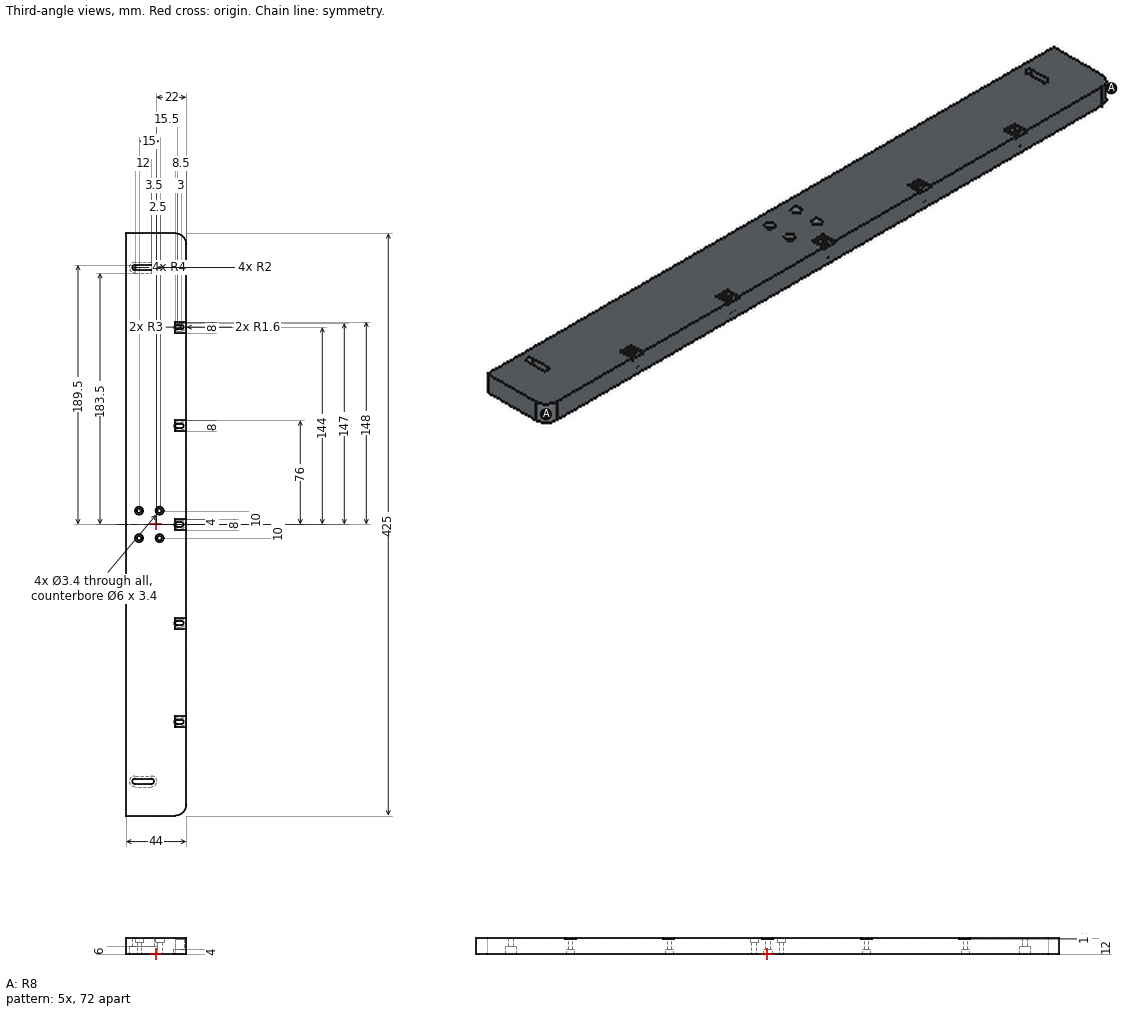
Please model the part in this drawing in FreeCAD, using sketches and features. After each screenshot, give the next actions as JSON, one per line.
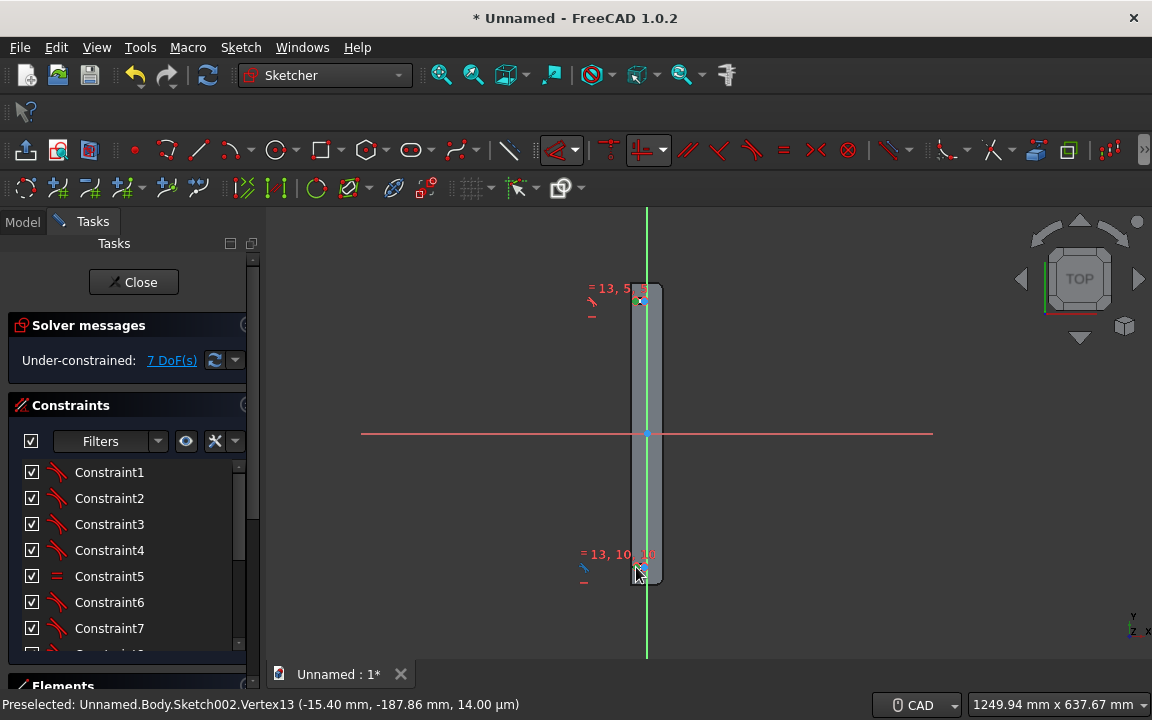
{"action": "left_click", "coordinate": [393, 434]}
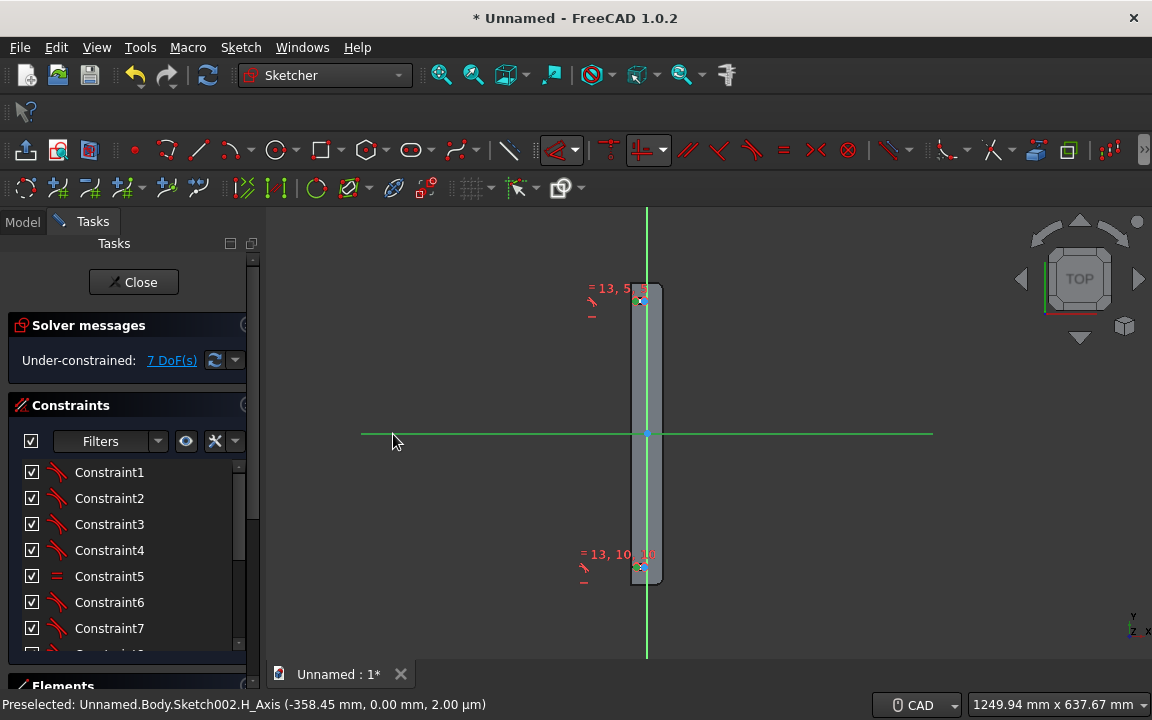
{"action": "key", "text": "s"}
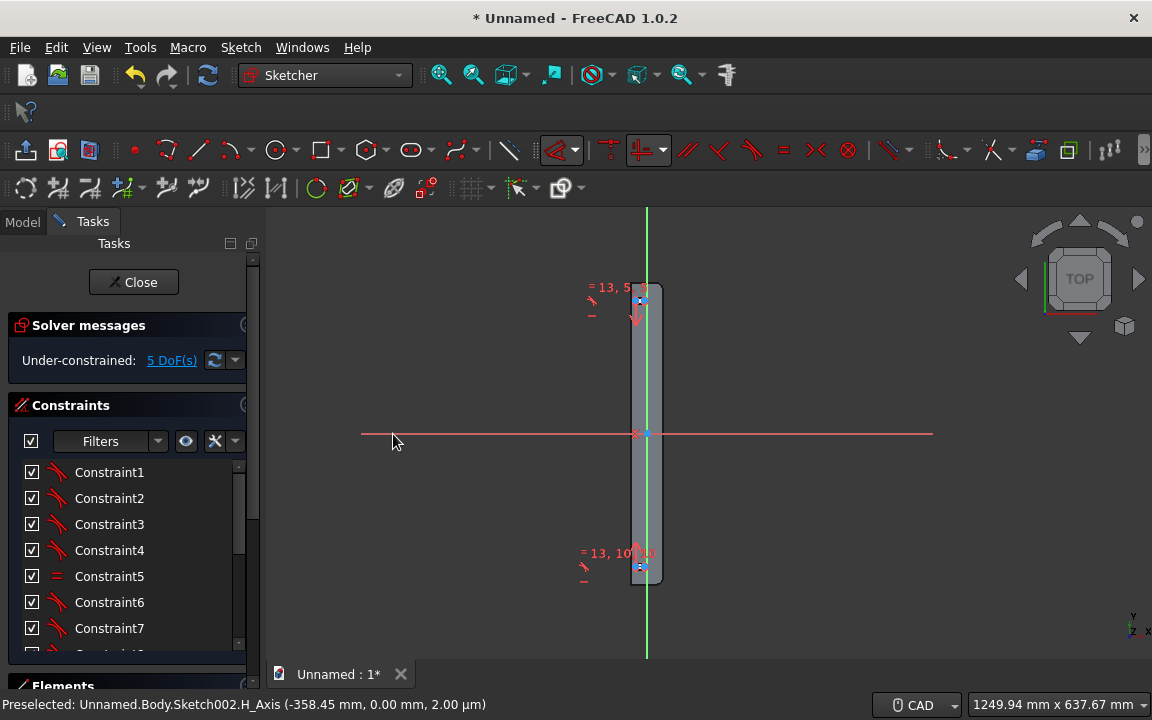
{"action": "scroll", "coordinate": [635, 301], "scroll_direction": "up", "scroll_amount": 17}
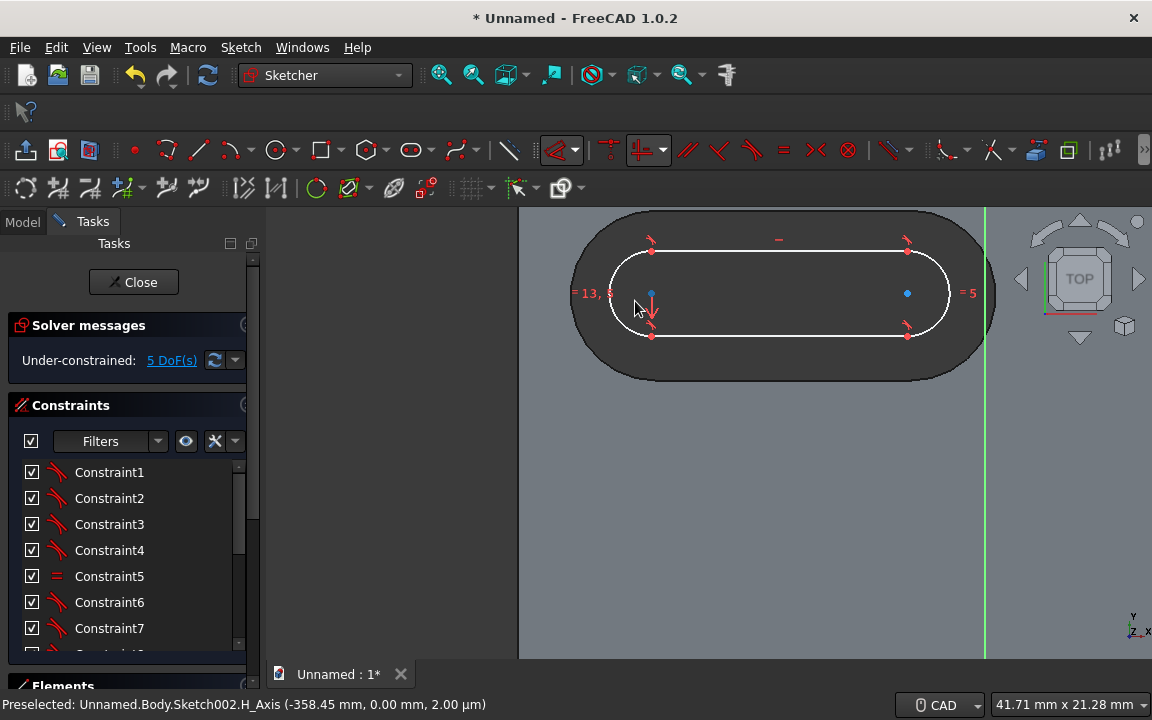
{"action": "left_click", "coordinate": [618, 269]}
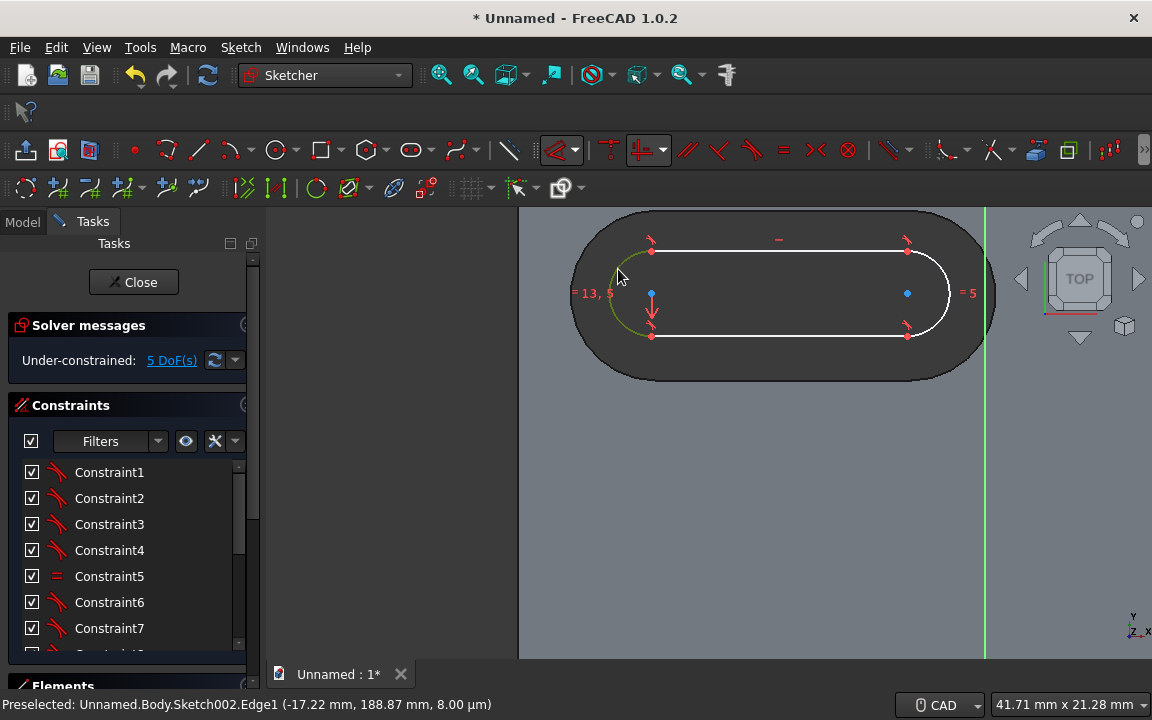
{"action": "key", "text": "k r"}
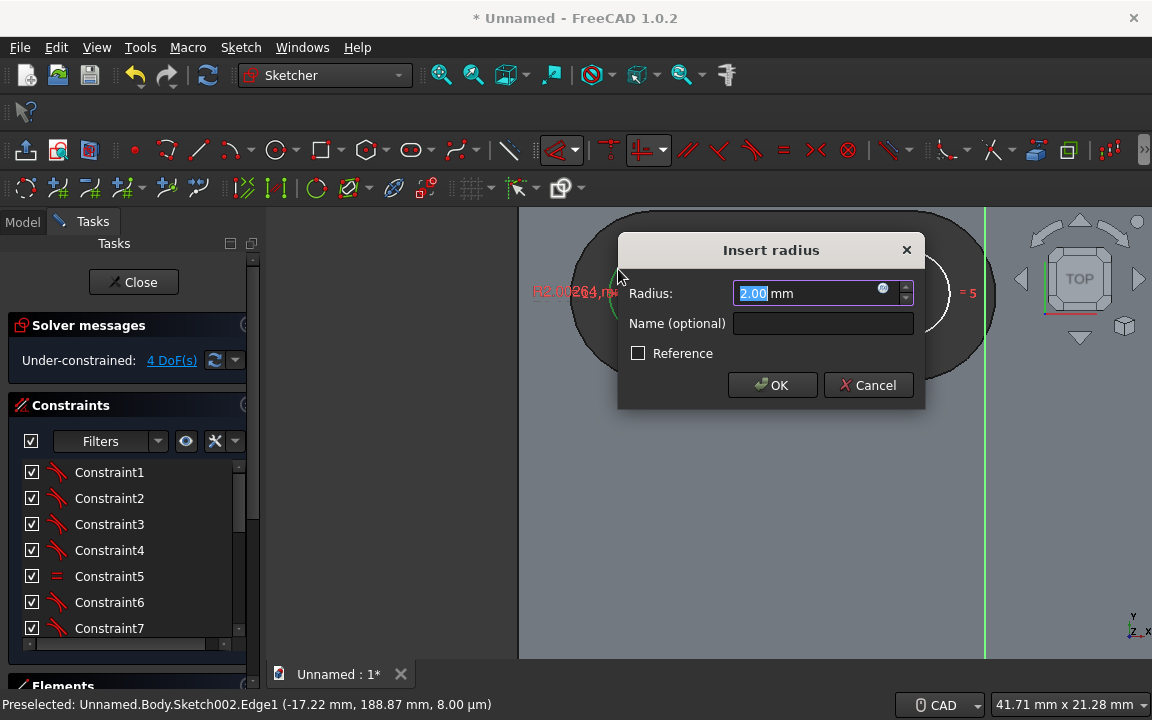
{"action": "type", "text": "2"}
{"action": "key", "text": "Return"}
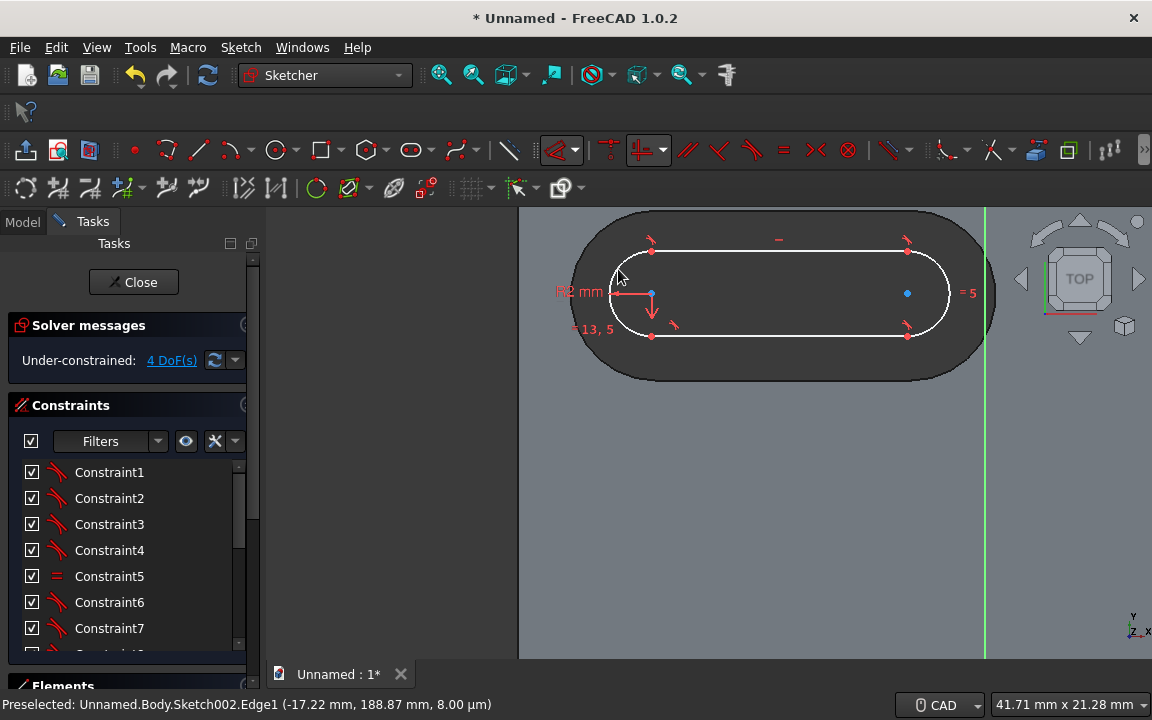
{"action": "scroll", "coordinate": [634, 270], "scroll_direction": "down", "scroll_amount": 16}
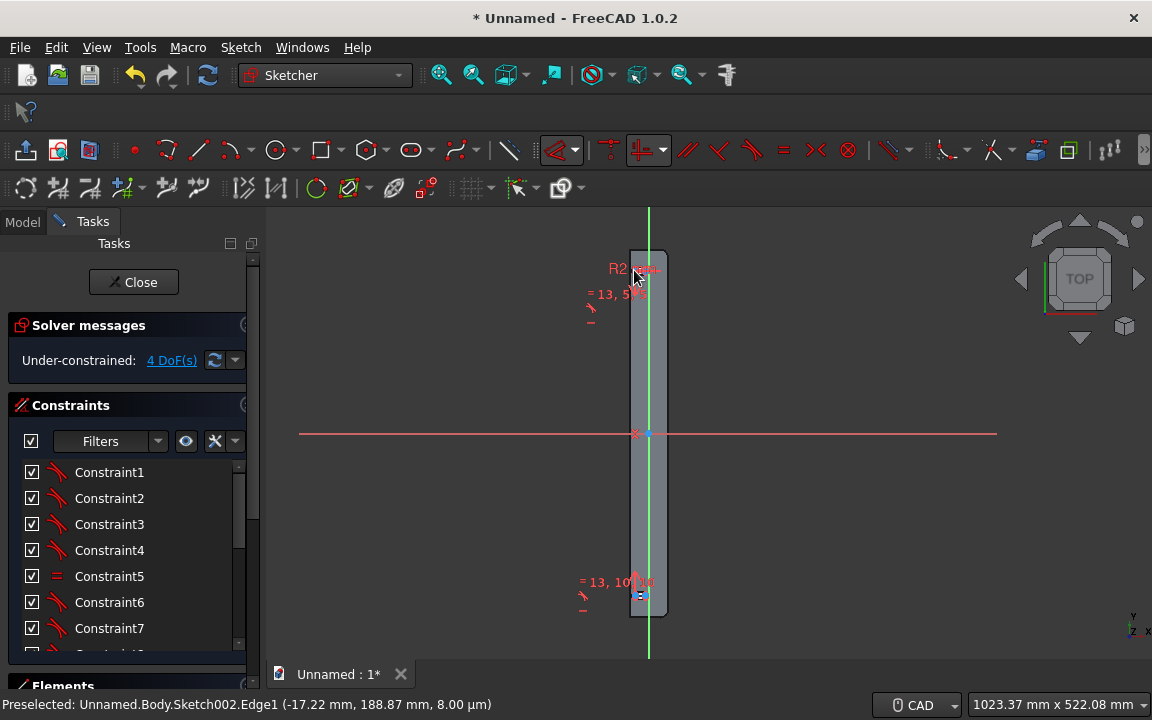
{"action": "scroll", "coordinate": [638, 269], "scroll_direction": "up", "scroll_amount": 8}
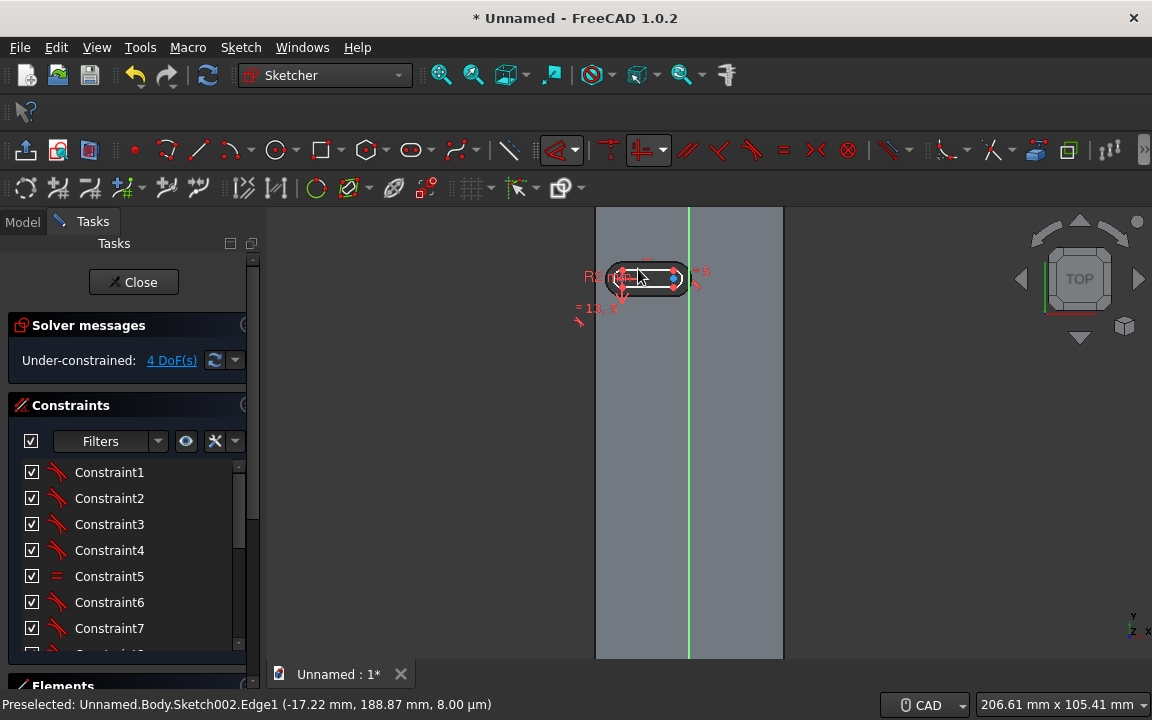
{"action": "left_click", "coordinate": [638, 270]}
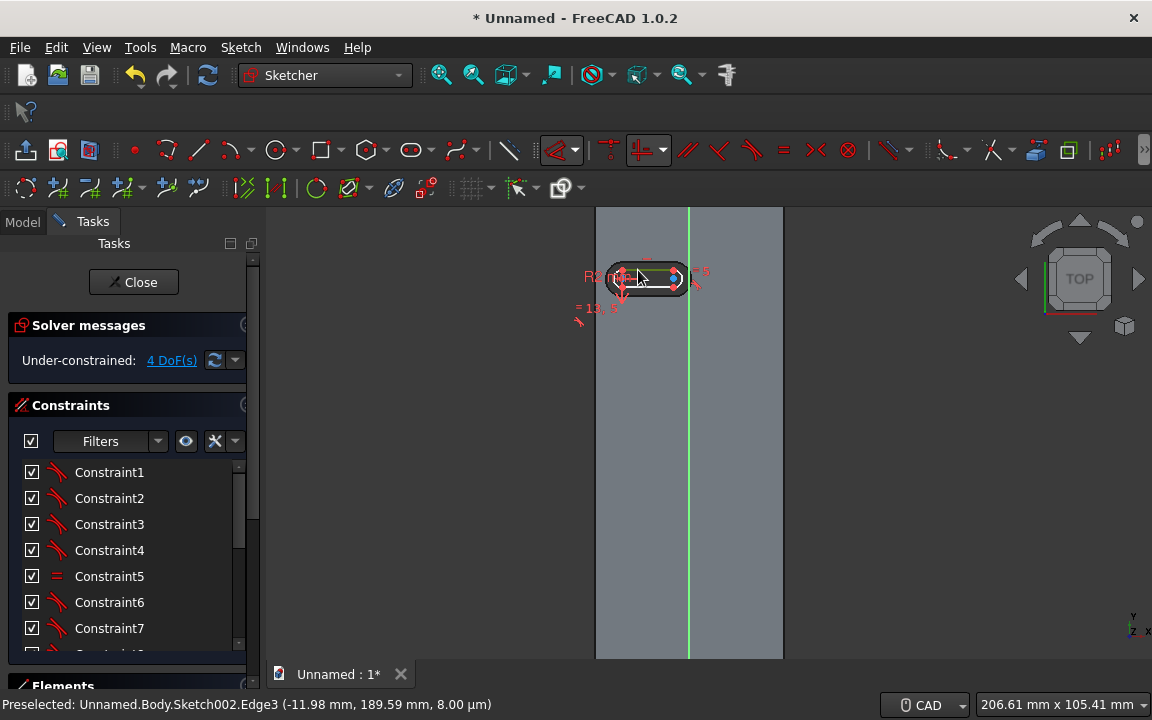
{"action": "left_click", "coordinate": [578, 150]}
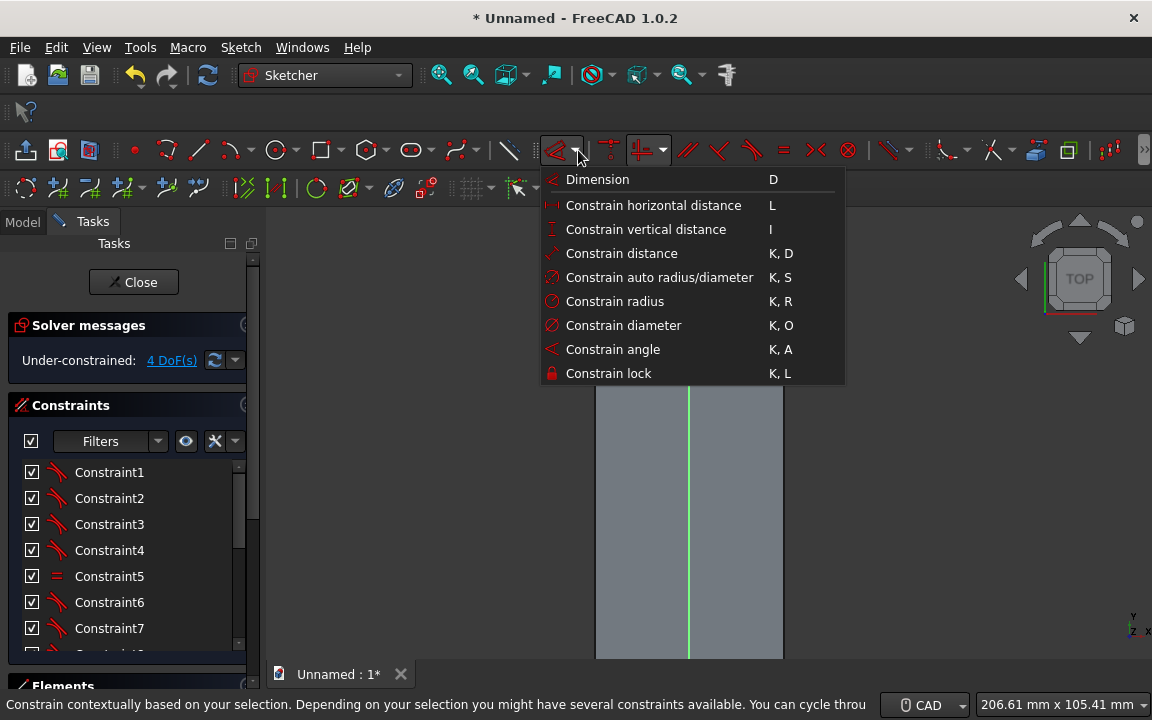
{"action": "left_click", "coordinate": [693, 205]}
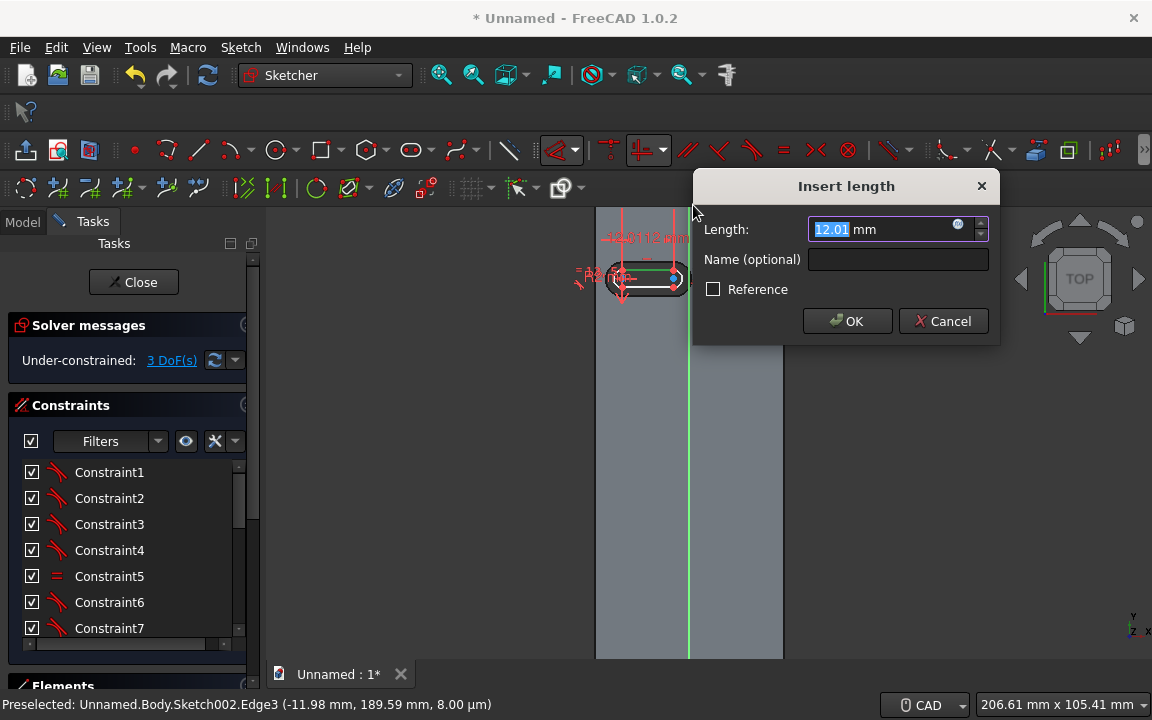
{"action": "type", "text": "12"}
{"action": "key", "text": "Return"}